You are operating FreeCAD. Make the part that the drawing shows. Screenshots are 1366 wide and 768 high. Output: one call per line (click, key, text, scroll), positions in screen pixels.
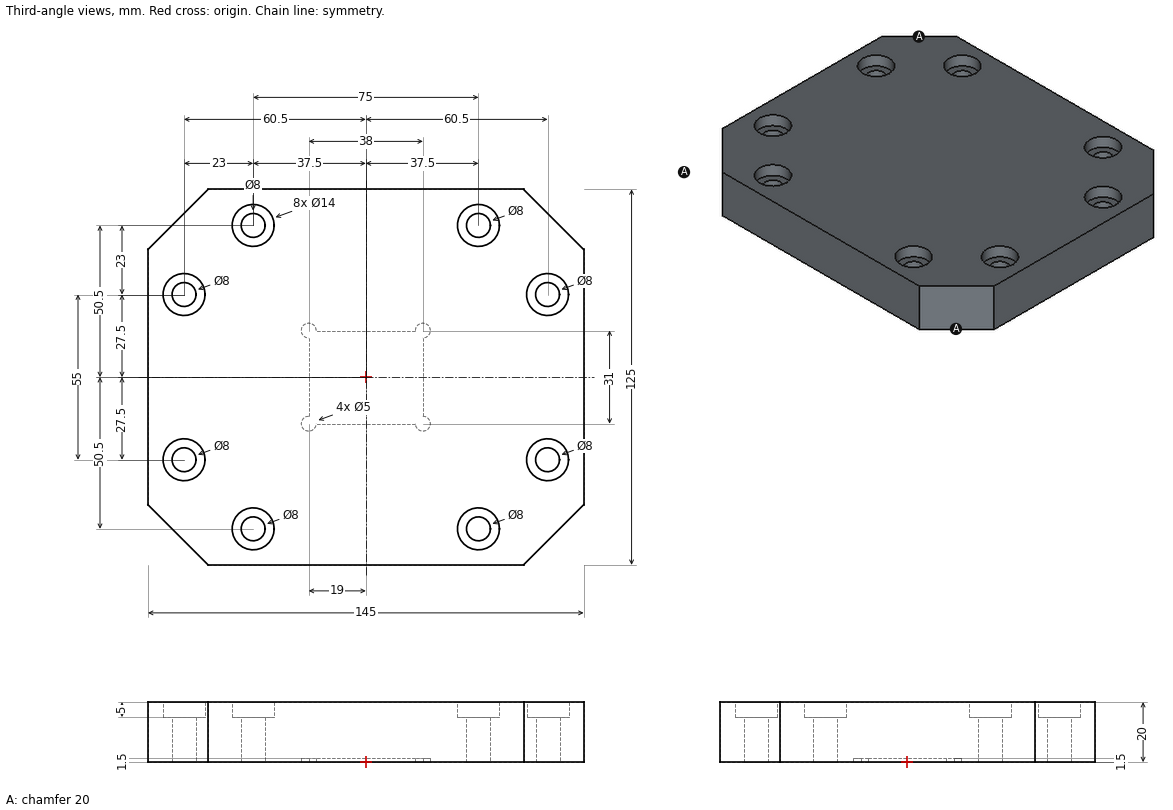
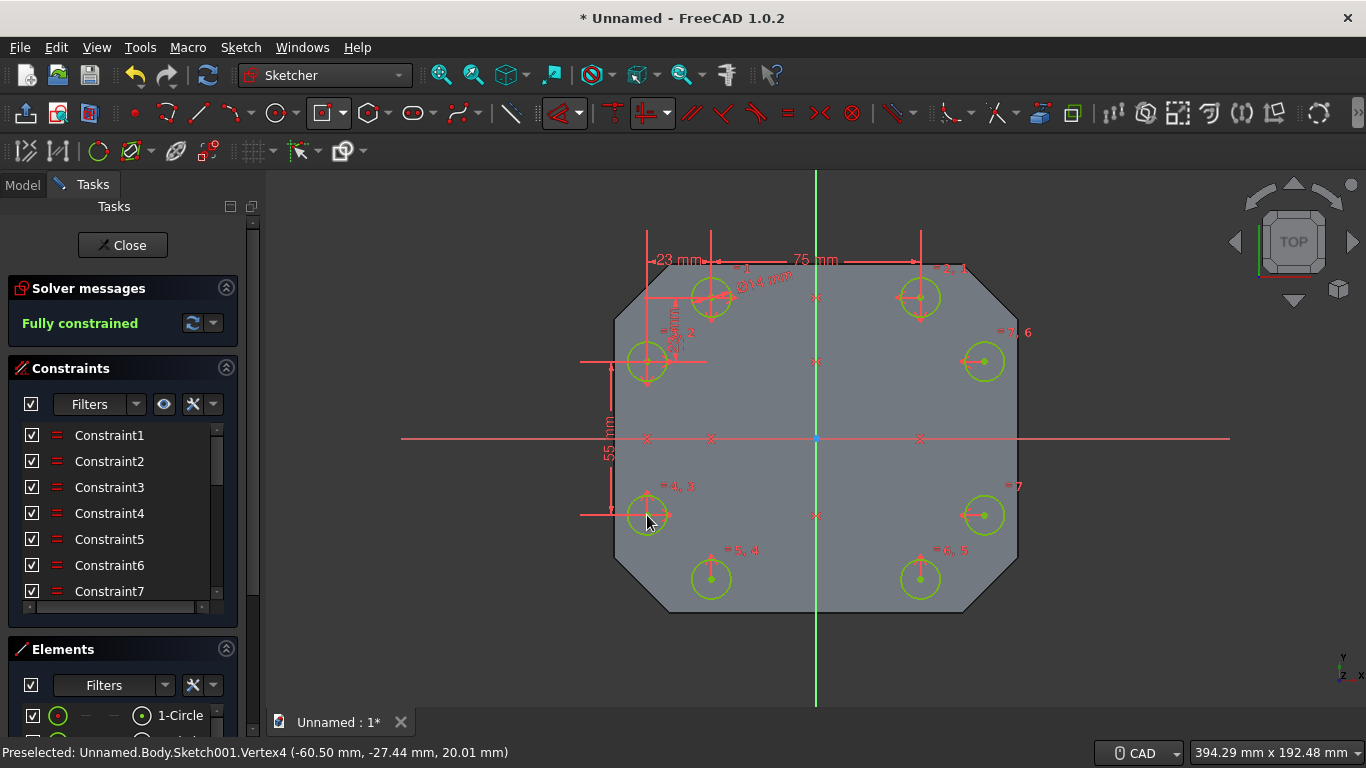
click(123, 245)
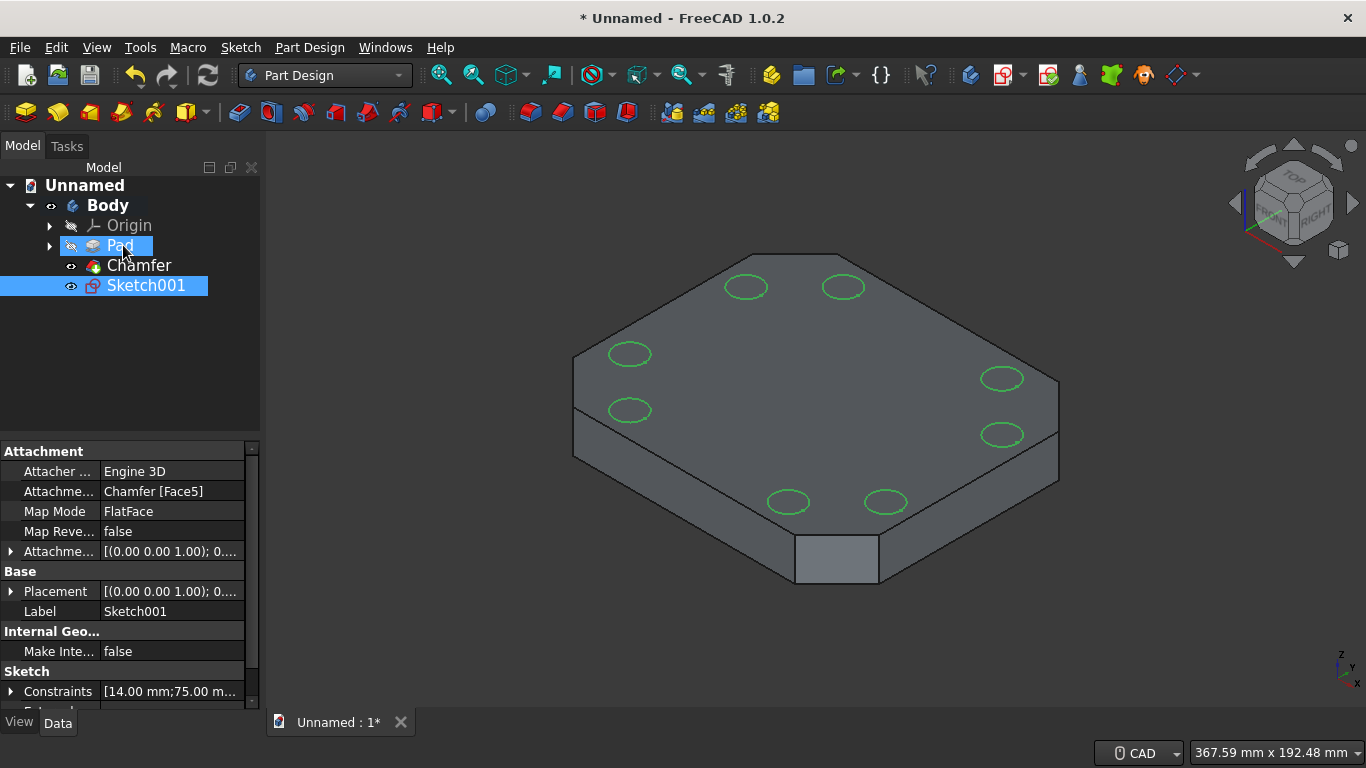
click(240, 112)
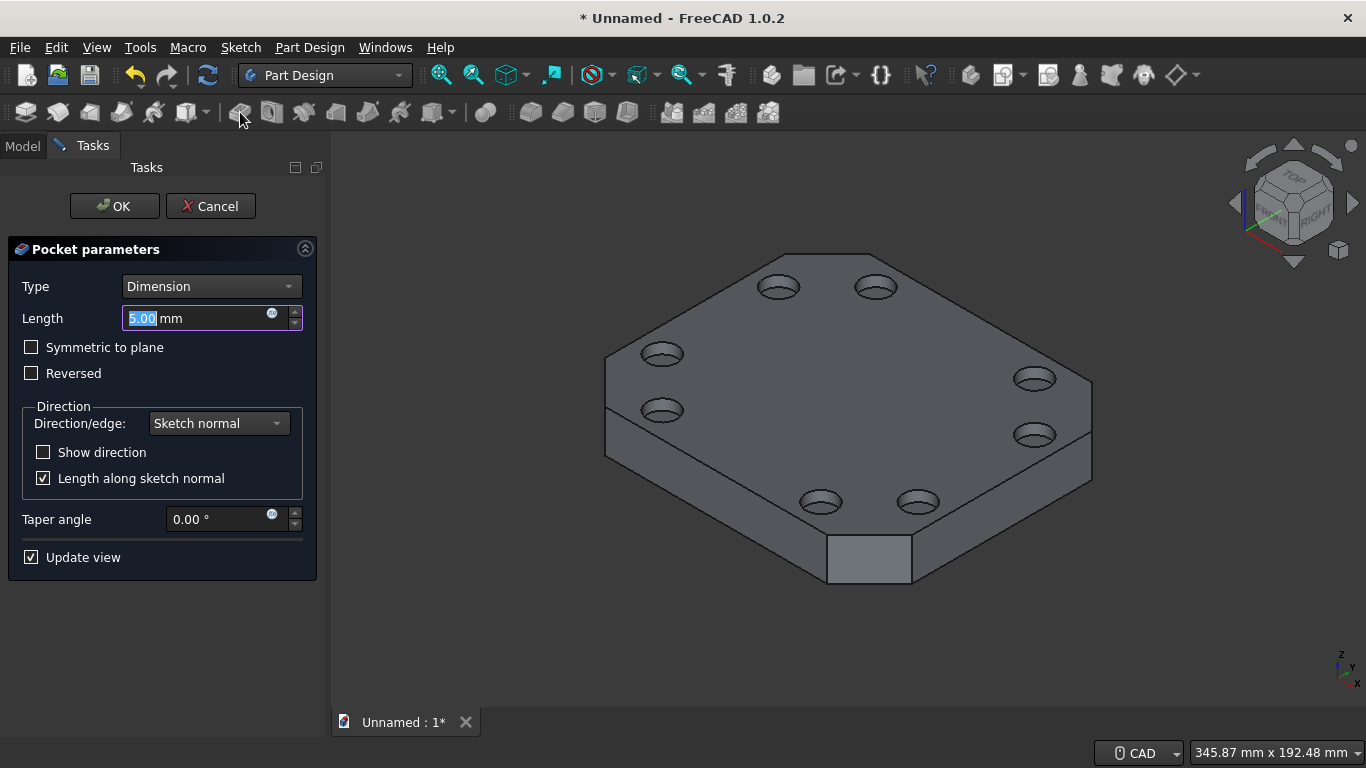
text(5)
key(Tab)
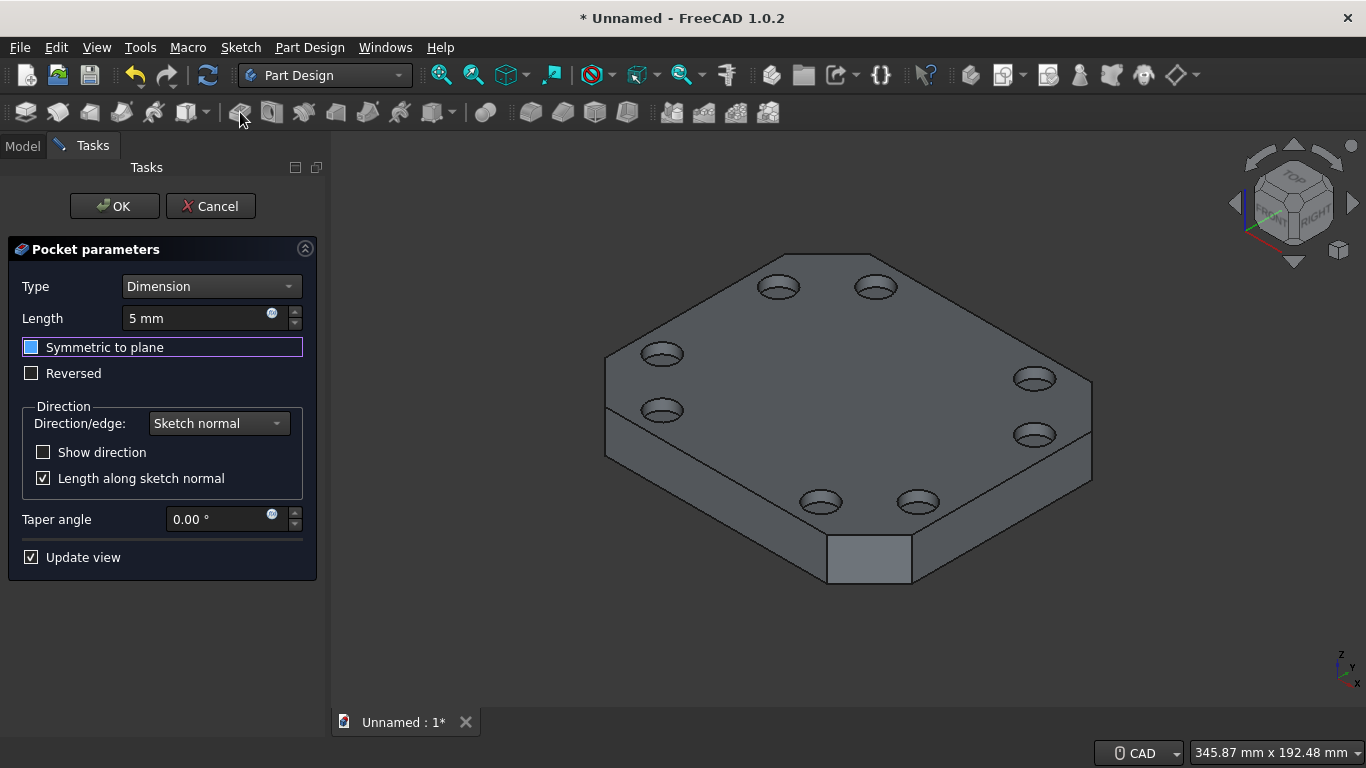
click(115, 206)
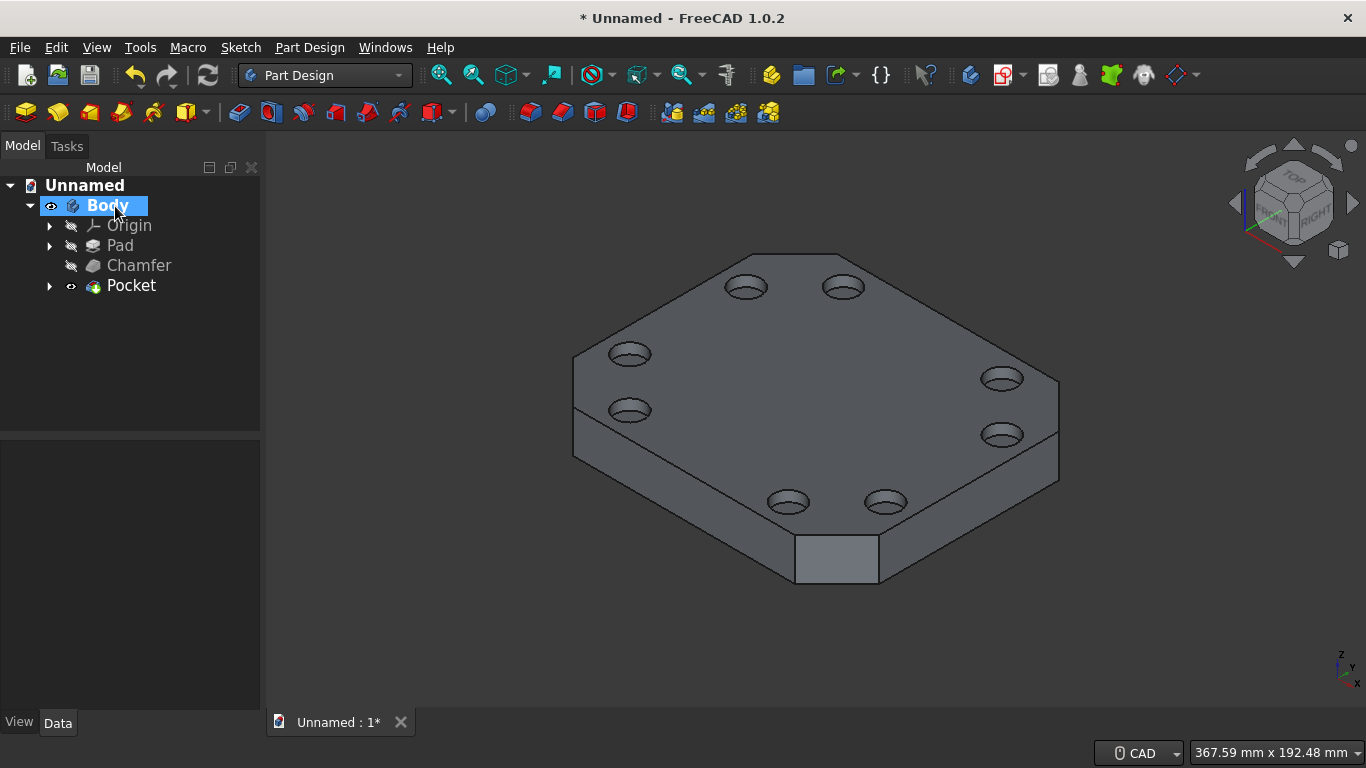
key(2)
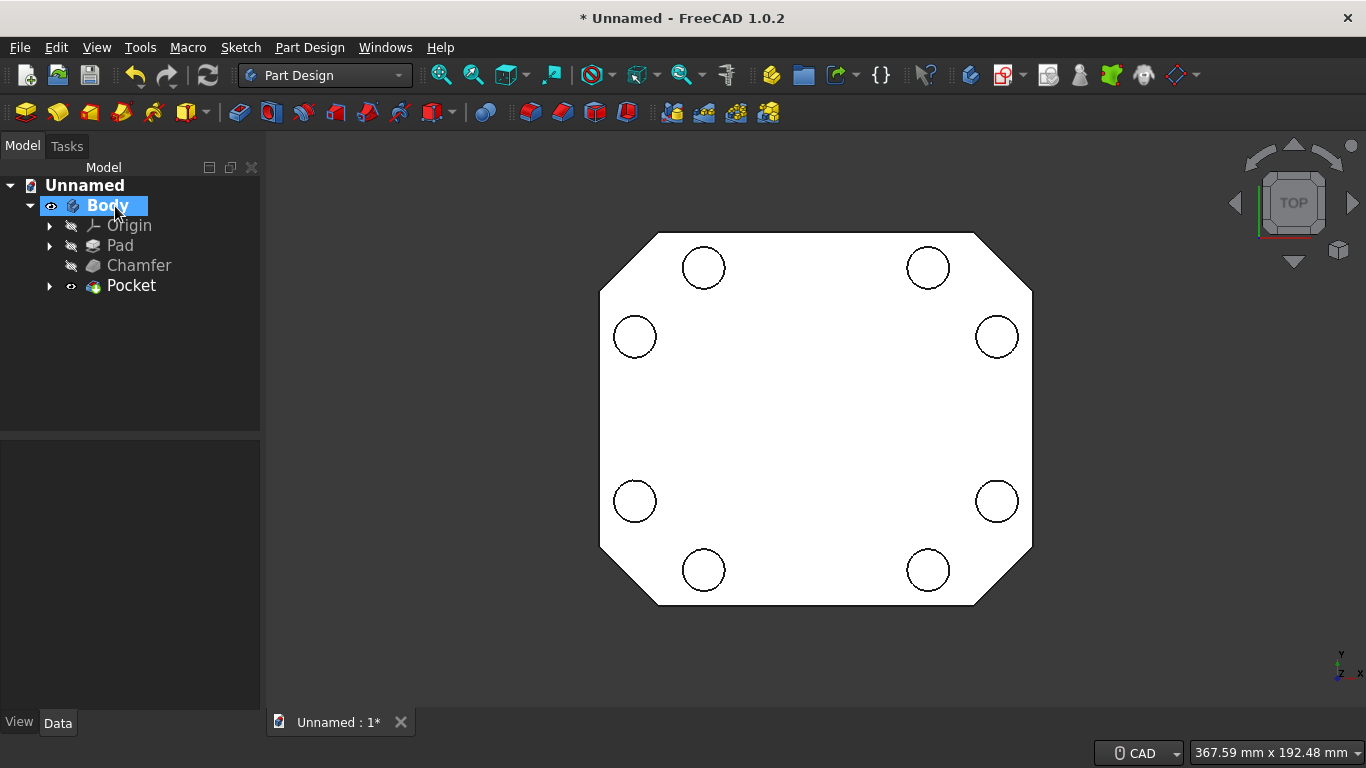
click(635, 336)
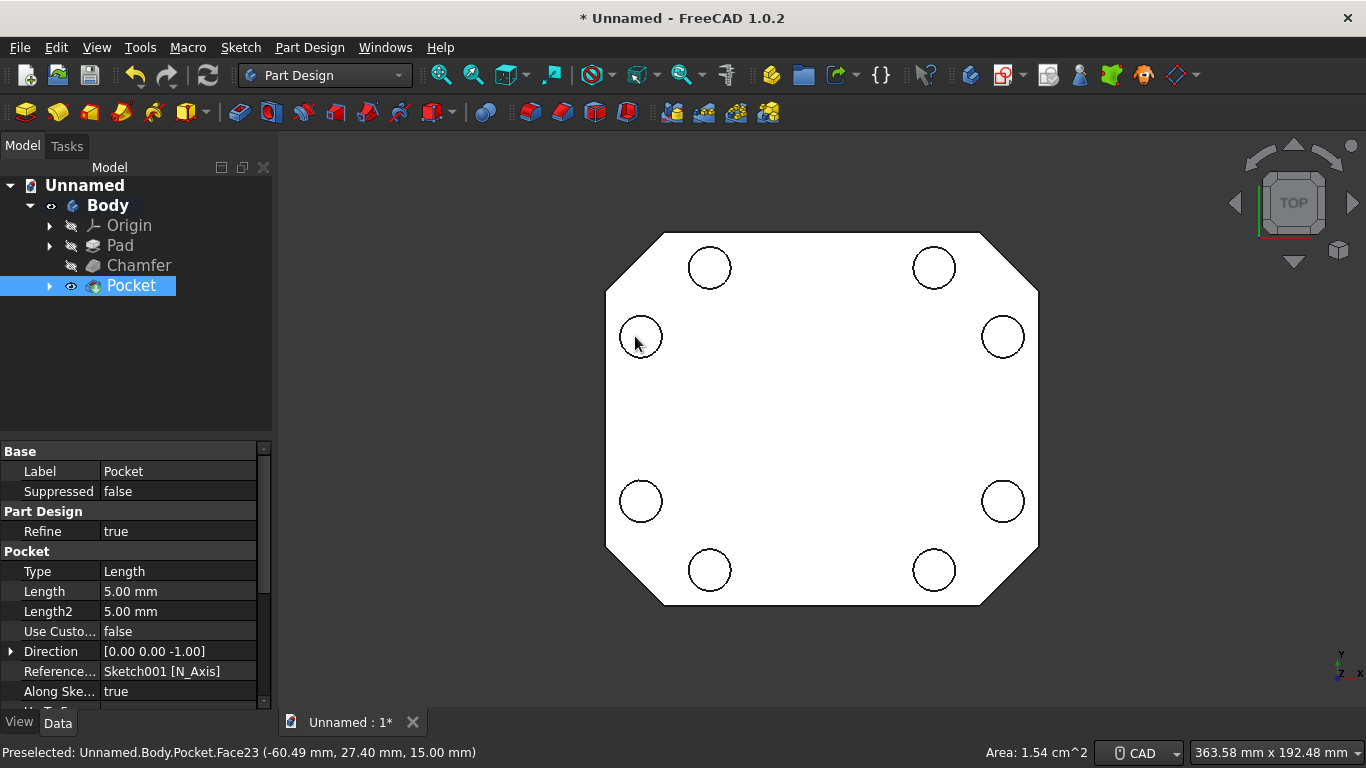
click(1004, 76)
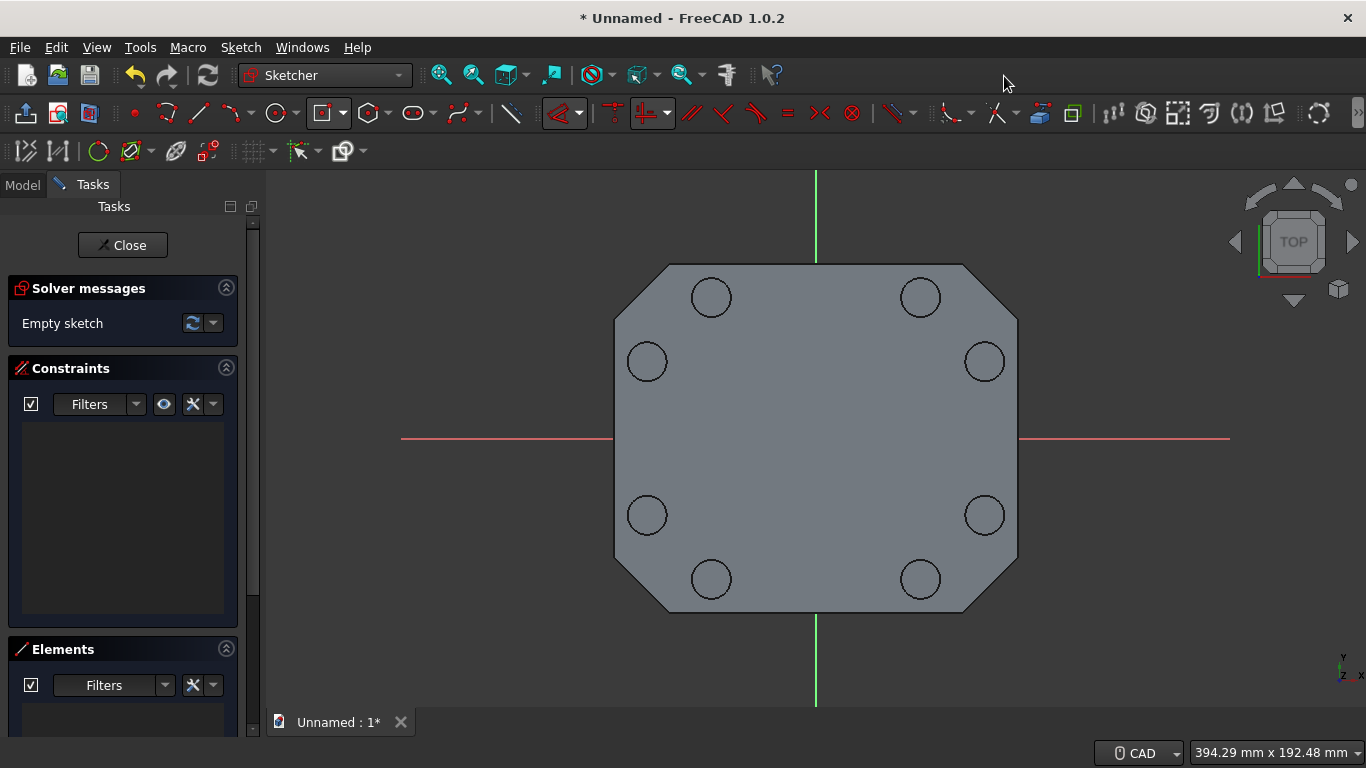
click(90, 114)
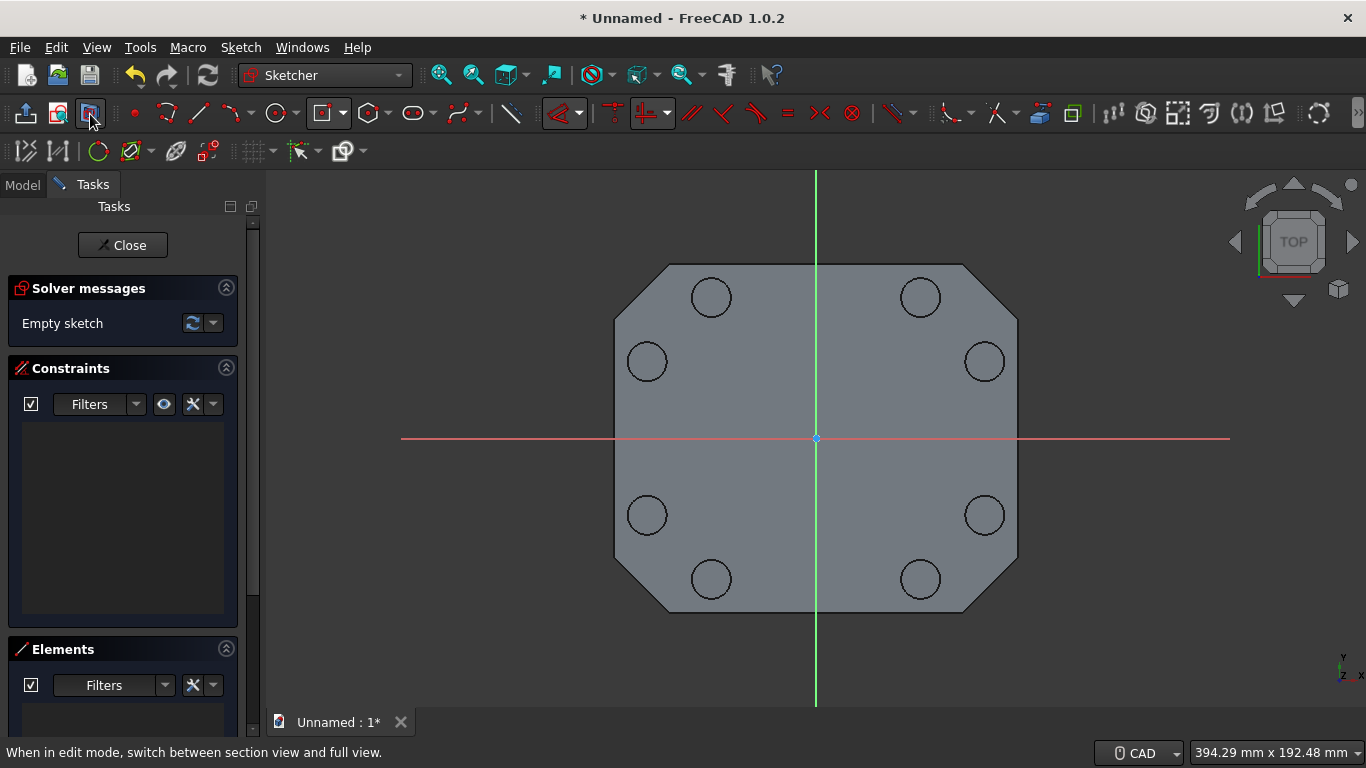
scroll(709, 288, up, 14)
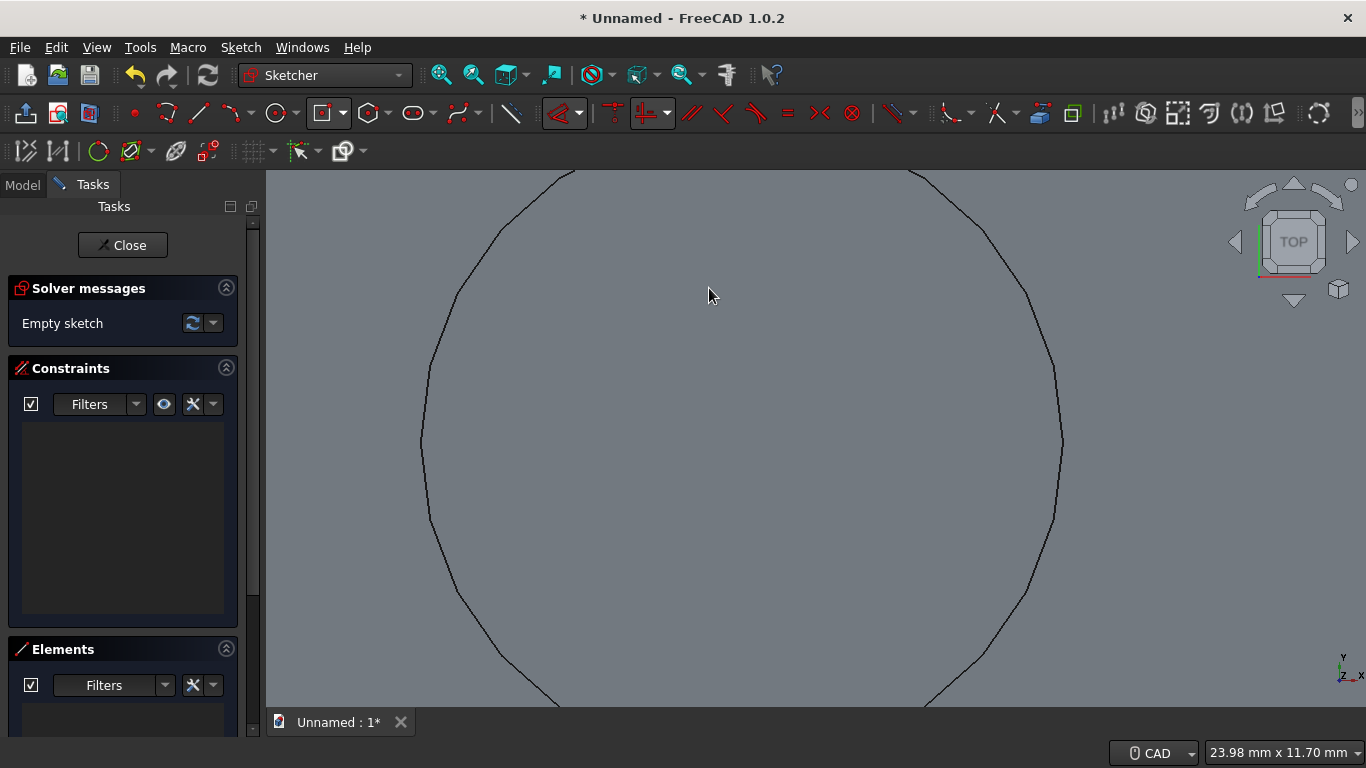
key(g)
key(c)